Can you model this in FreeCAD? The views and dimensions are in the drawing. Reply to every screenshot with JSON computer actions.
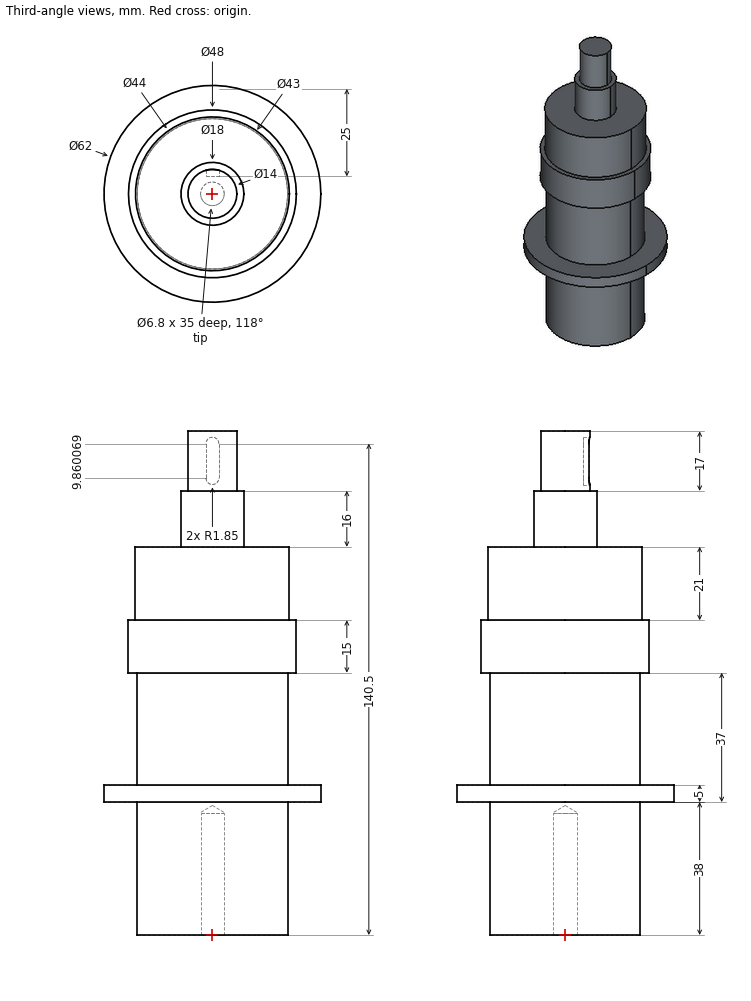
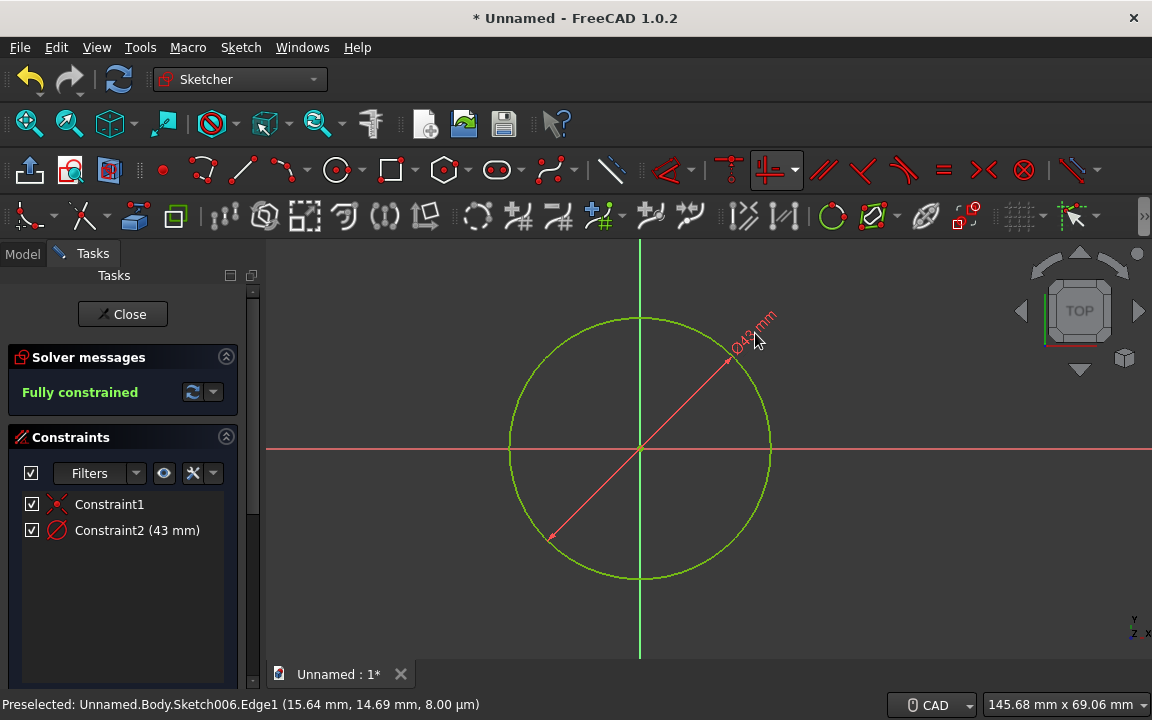
{"action": "left_click", "coordinate": [123, 314]}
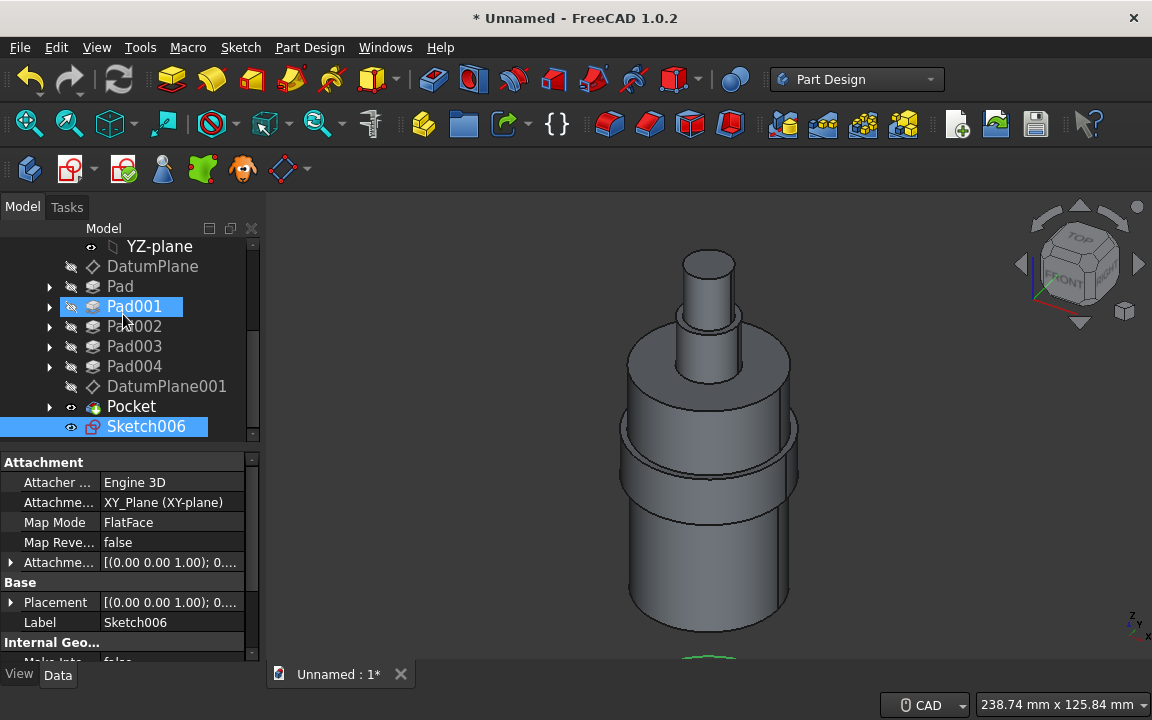
{"action": "left_click", "coordinate": [172, 80]}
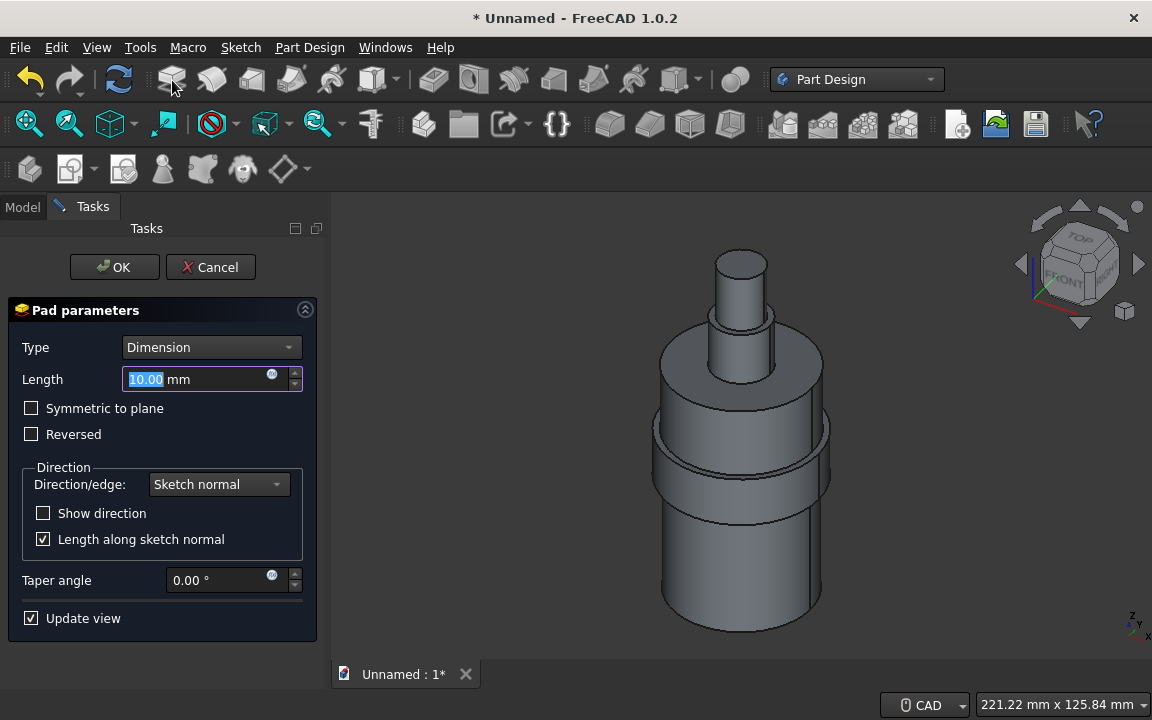
{"action": "type", "text": "38"}
{"action": "key", "text": "Tab"}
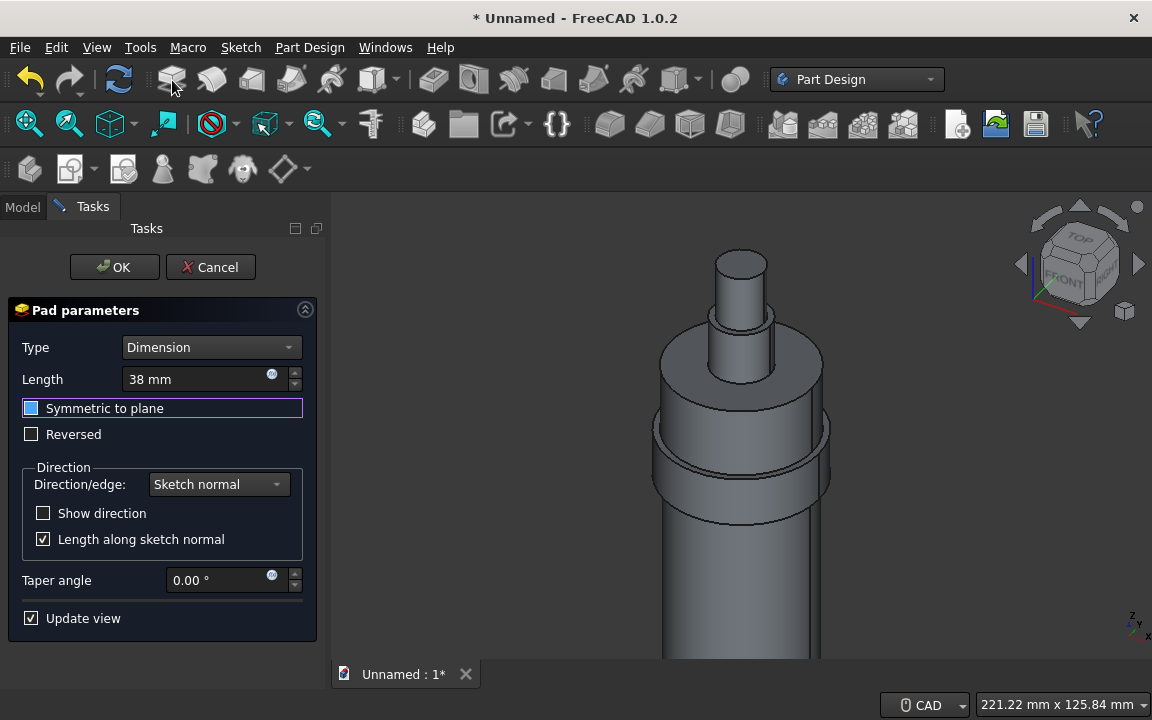
{"action": "left_click", "coordinate": [115, 267]}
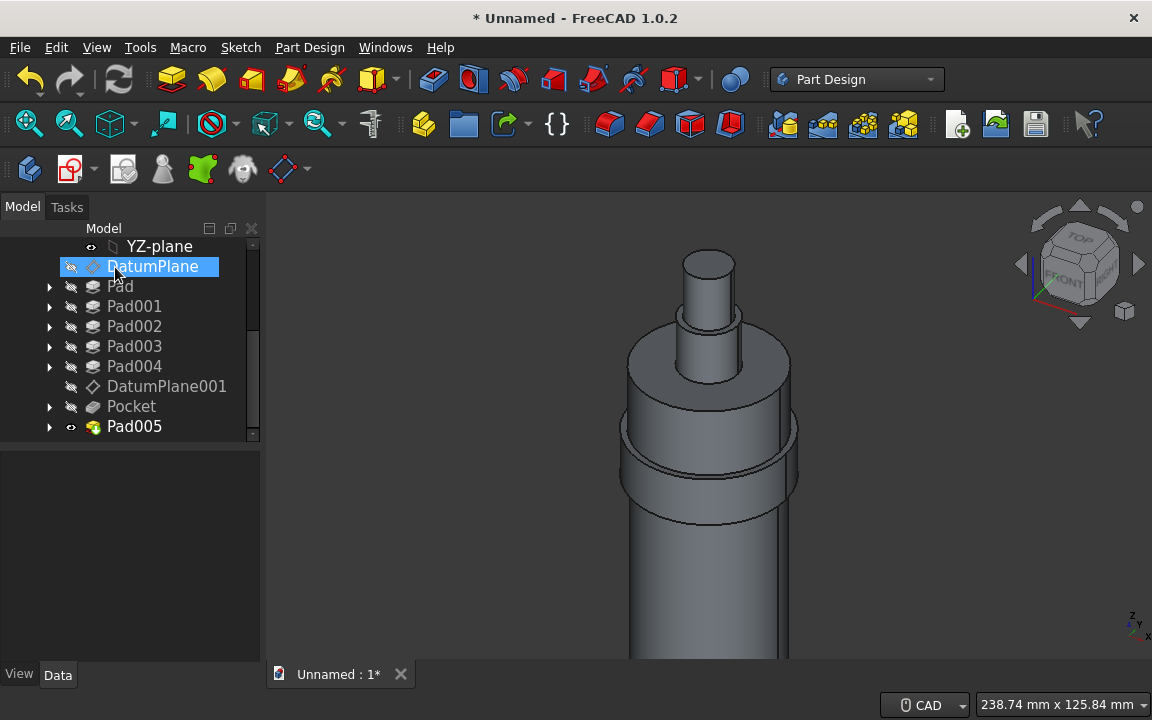
{"action": "left_click", "coordinate": [30, 124]}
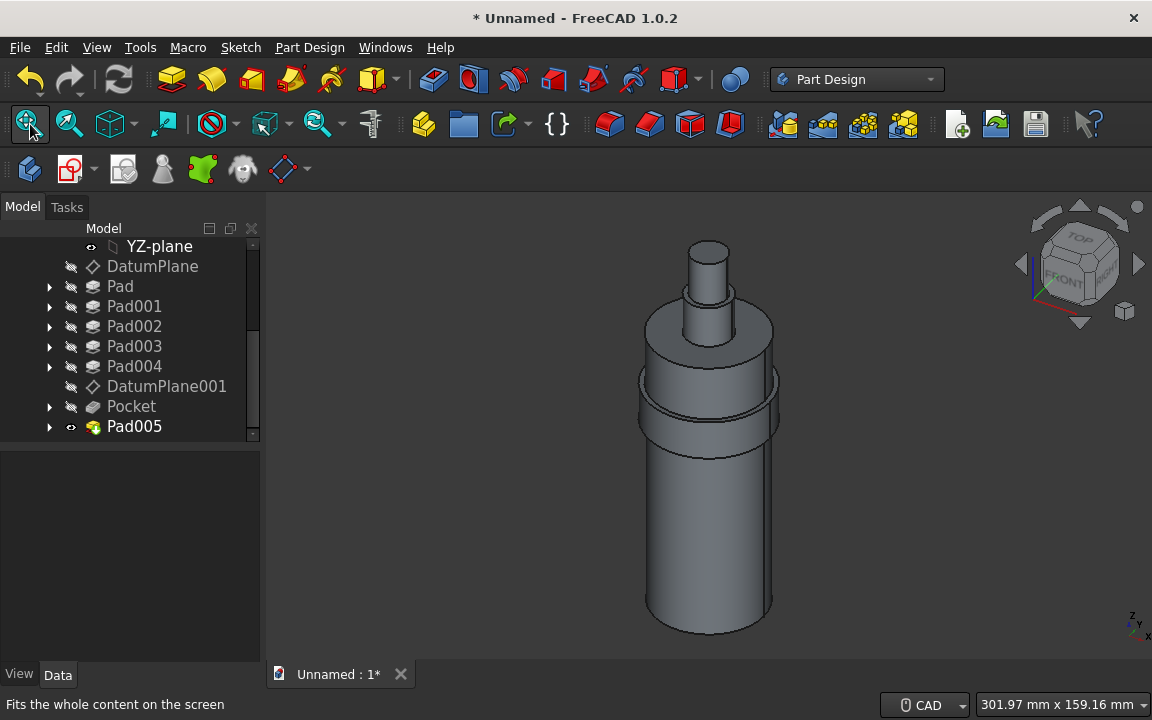
{"action": "scroll", "coordinate": [160, 342], "scroll_direction": "down", "scroll_amount": 3}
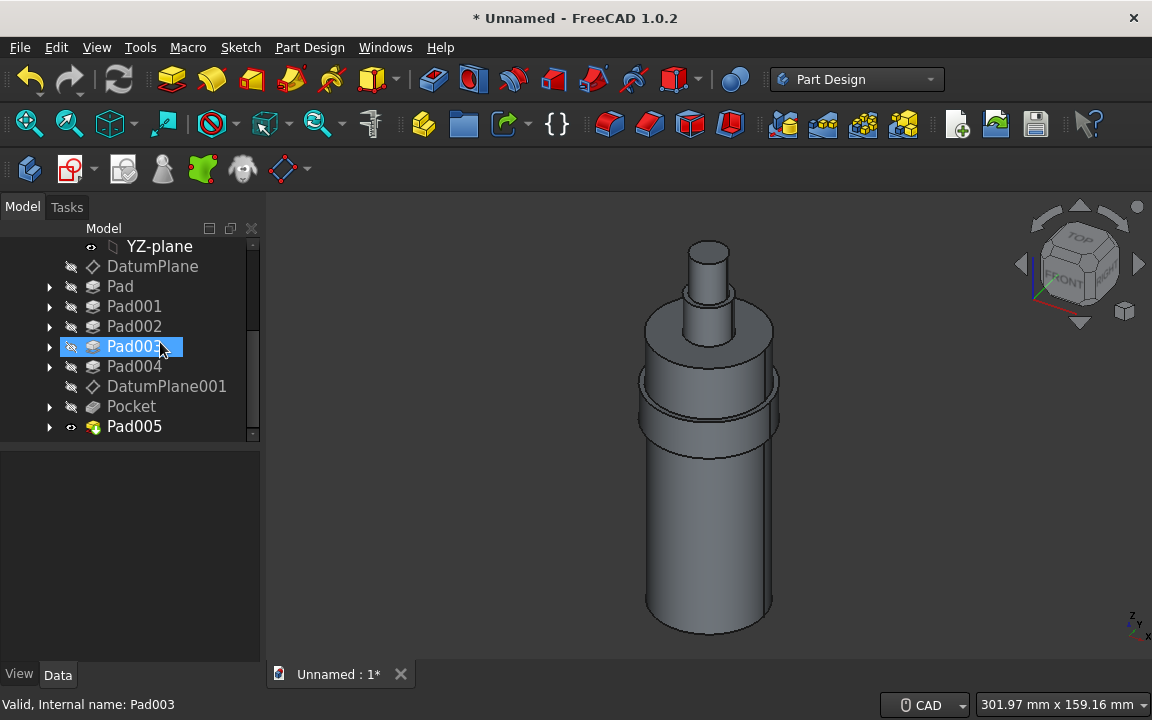
{"action": "scroll", "coordinate": [160, 342], "scroll_direction": "up", "scroll_amount": 15}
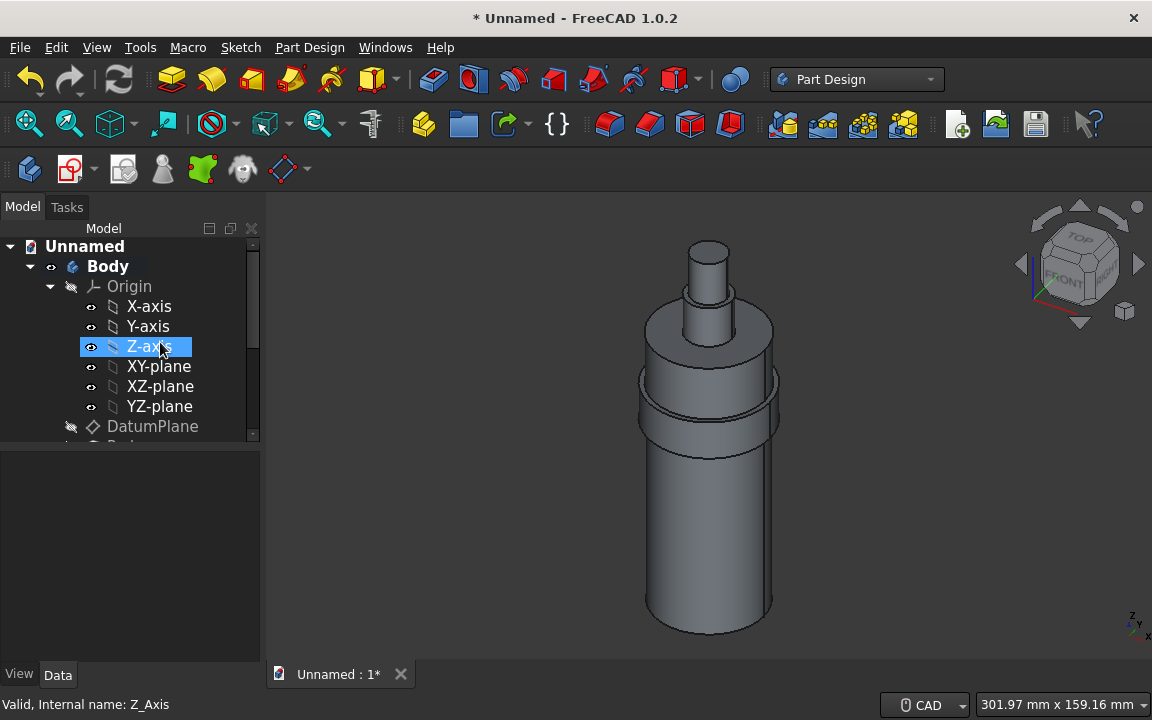
{"action": "left_click", "coordinate": [136, 367]}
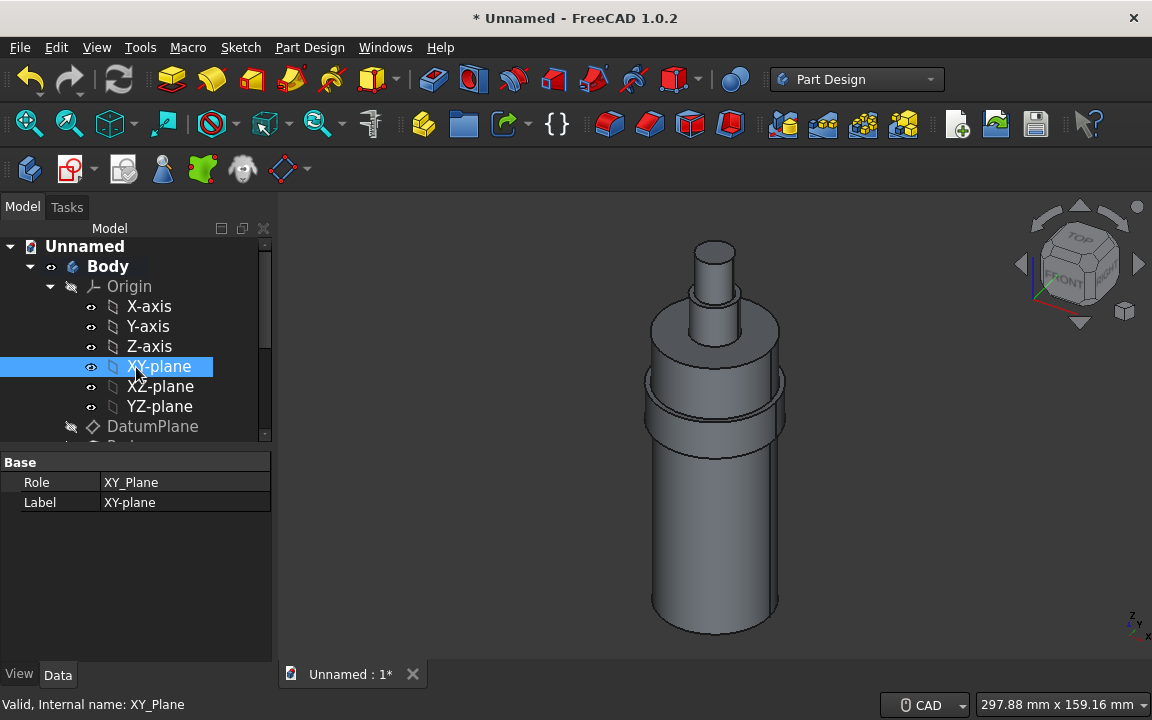
{"action": "left_click", "coordinate": [284, 170]}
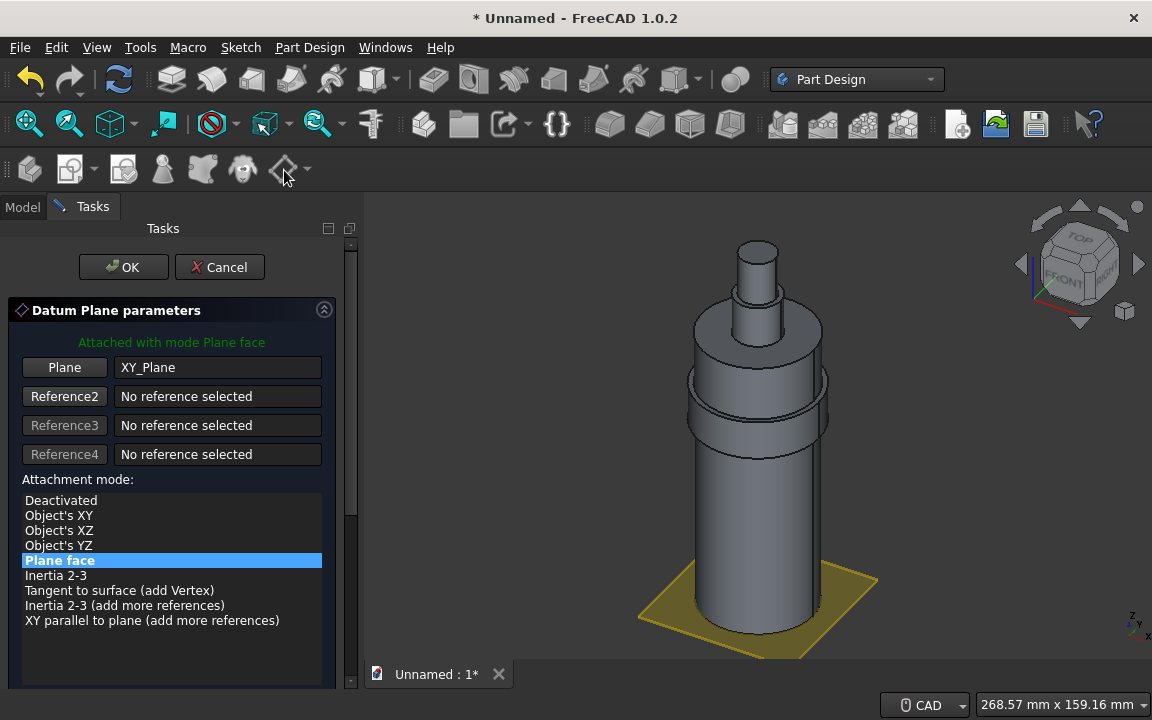
{"action": "scroll", "coordinate": [351, 463], "scroll_direction": "down", "scroll_amount": 3}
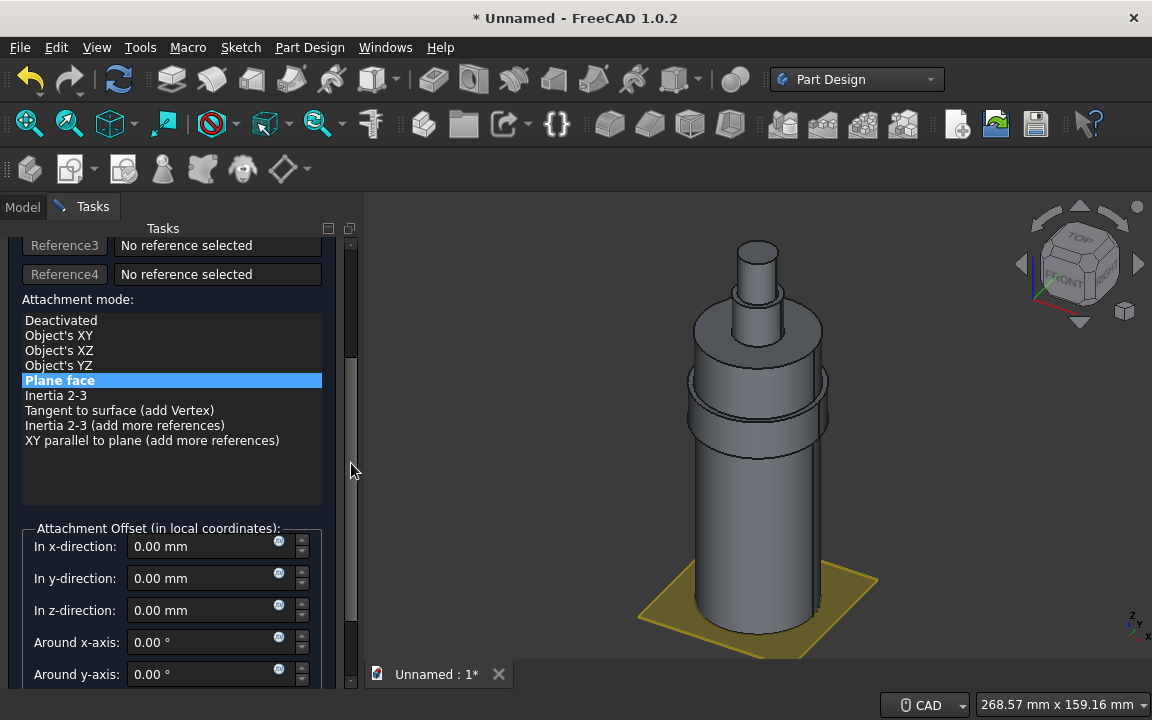
{"action": "triple_click", "coordinate": [210, 610]}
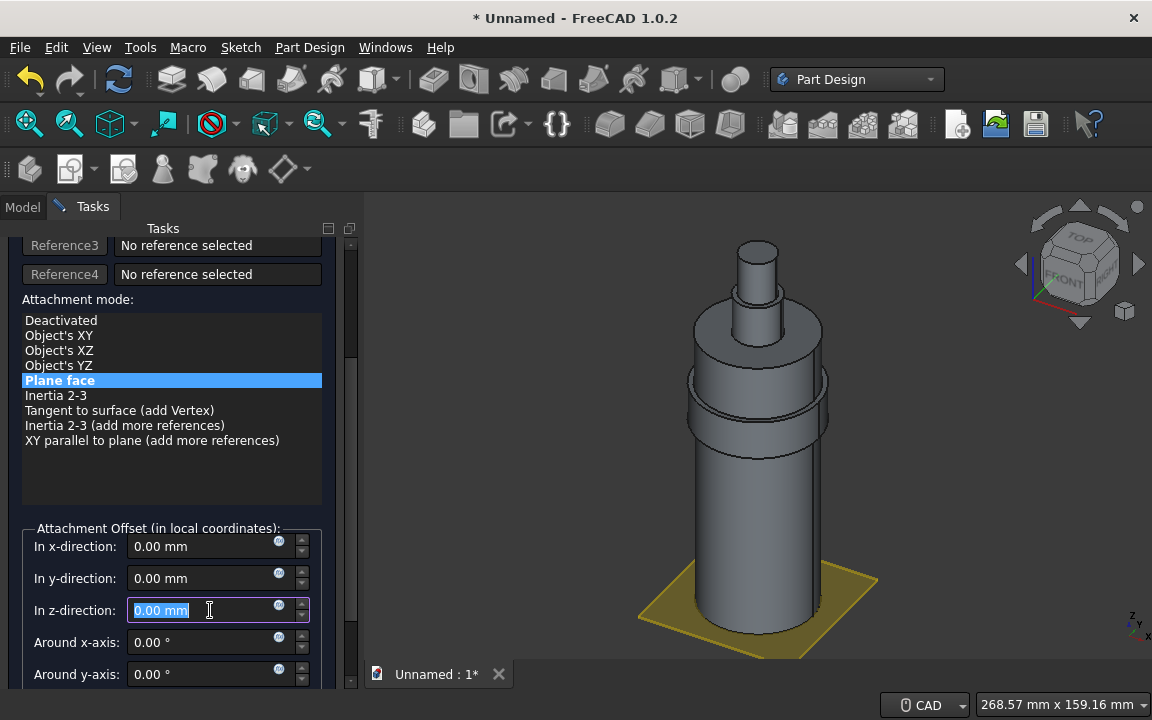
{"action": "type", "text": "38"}
{"action": "key", "text": "Tab"}